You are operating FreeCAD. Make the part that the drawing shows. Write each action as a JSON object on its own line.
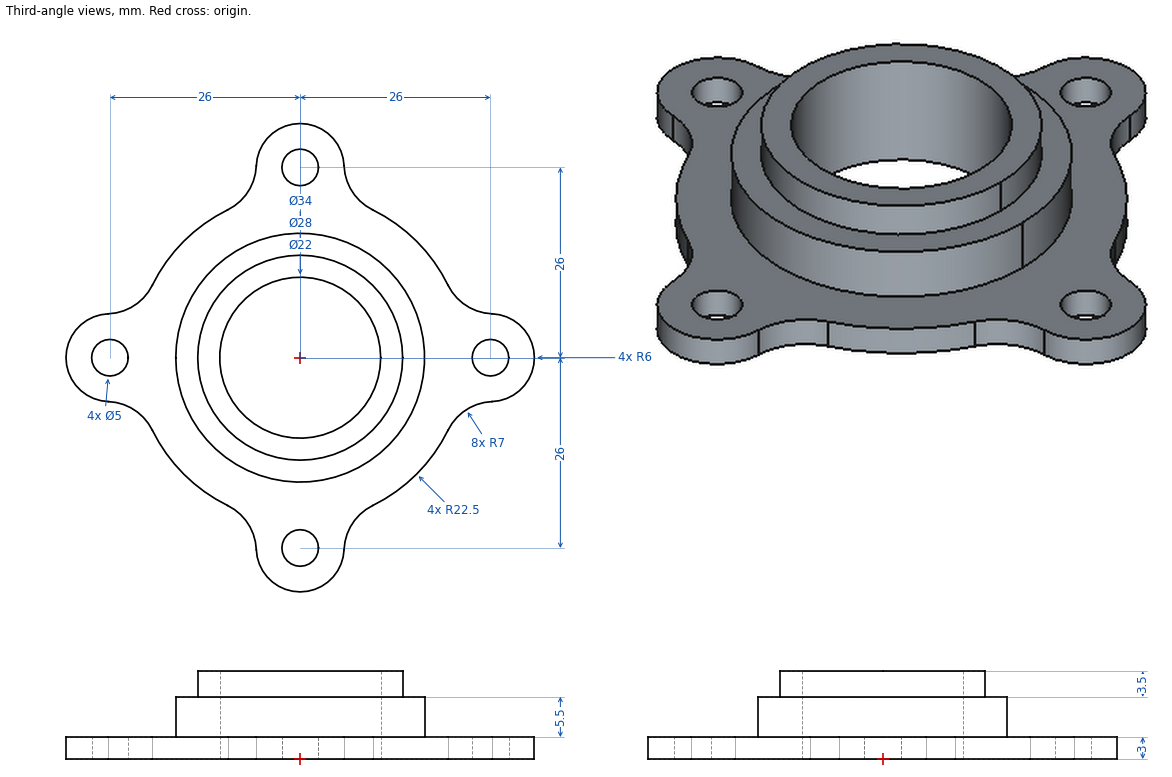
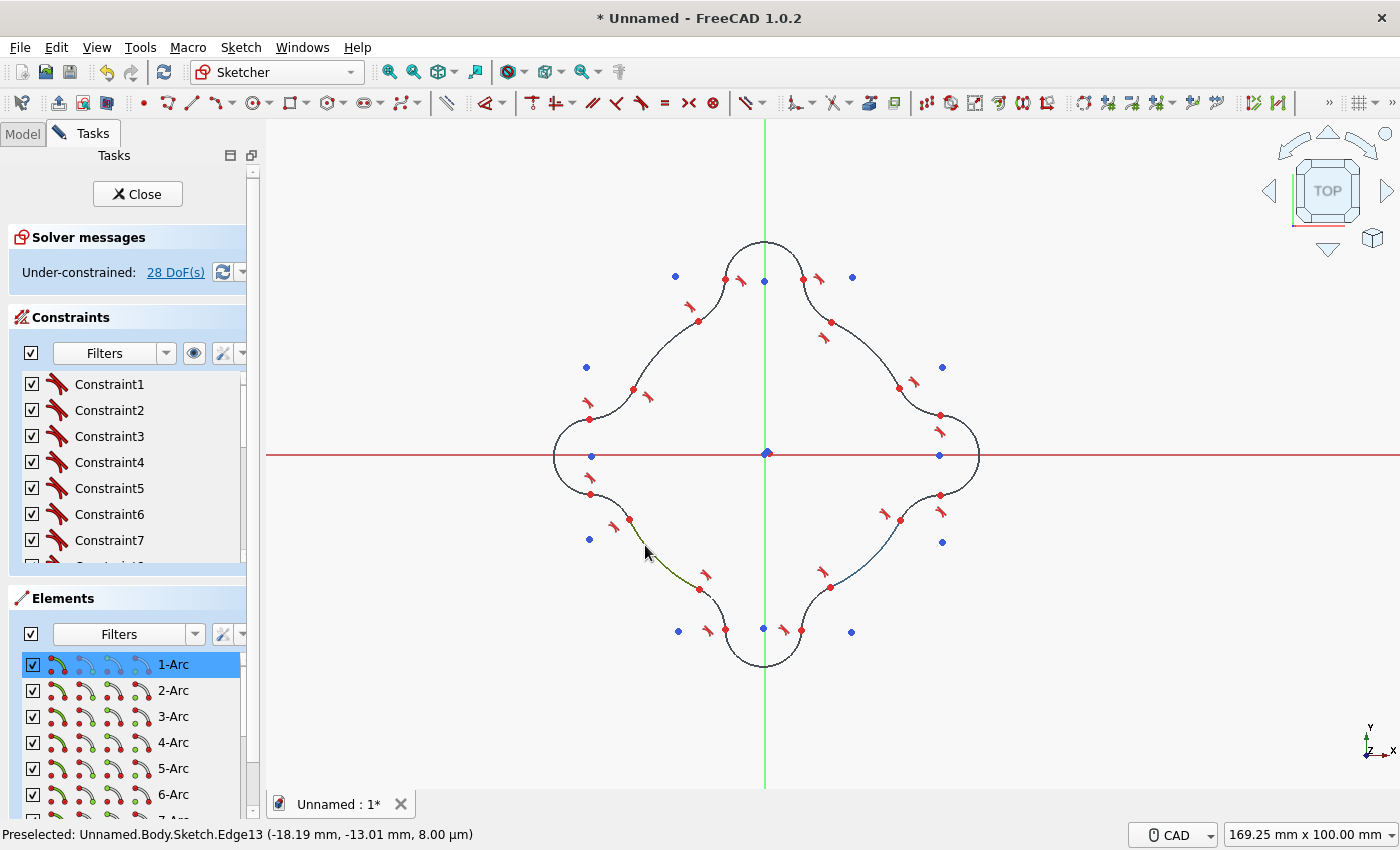
{"action": "left_click", "coordinate": [532, 104]}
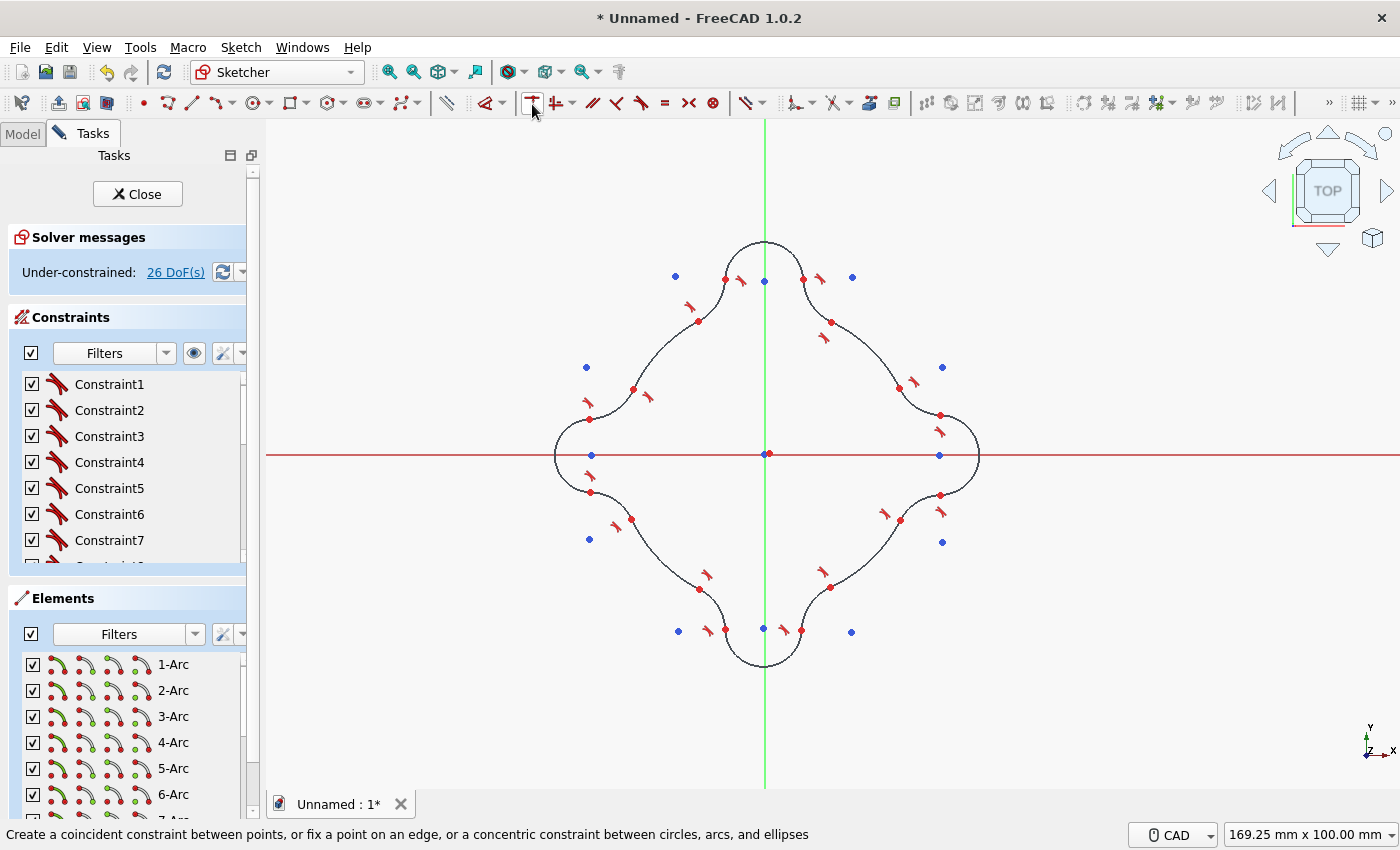
{"action": "left_click_drag", "start_coordinate": [755, 444], "coordinate": [780, 465]}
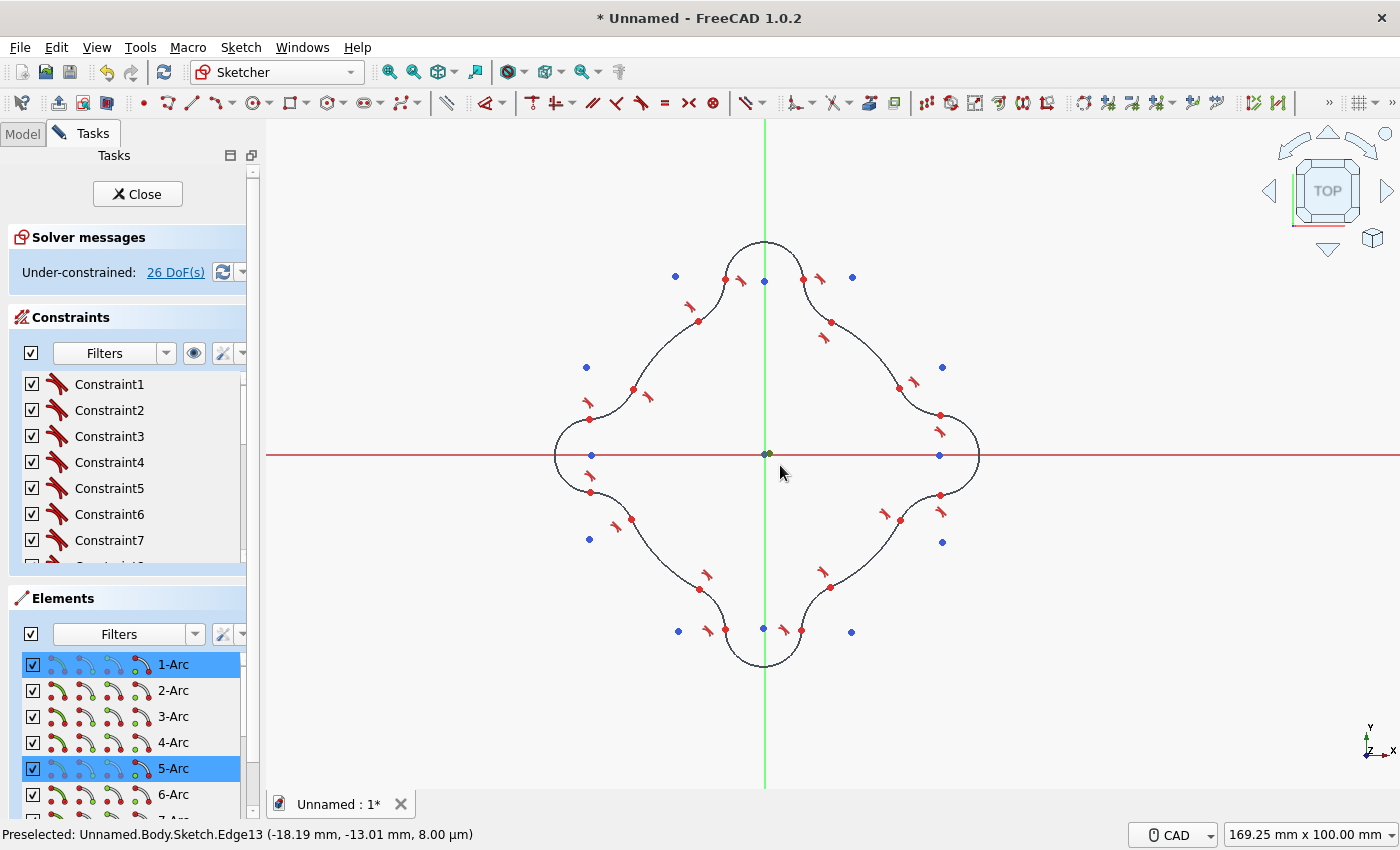
{"action": "left_click", "coordinate": [532, 104]}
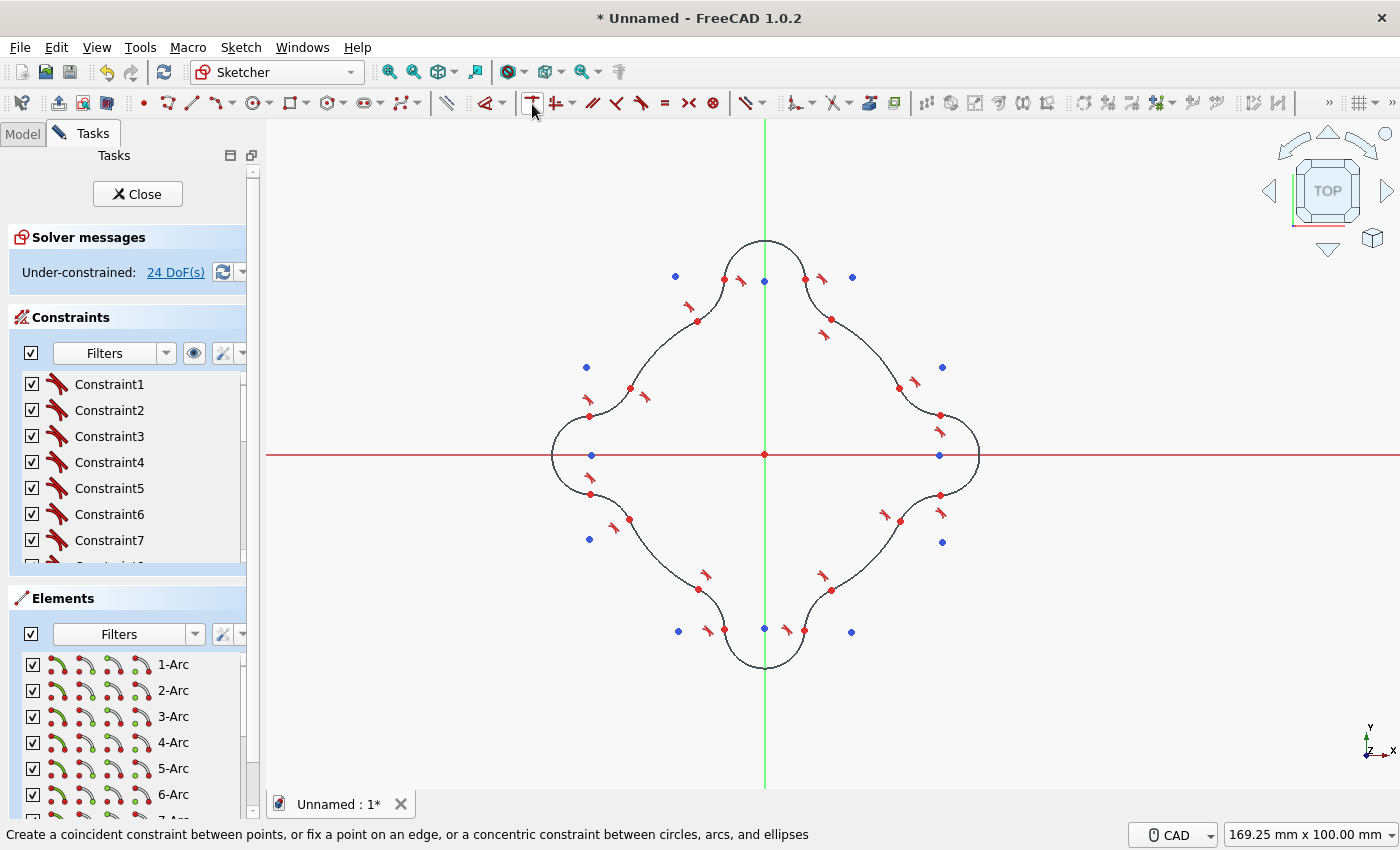
{"action": "left_click", "coordinate": [926, 498]}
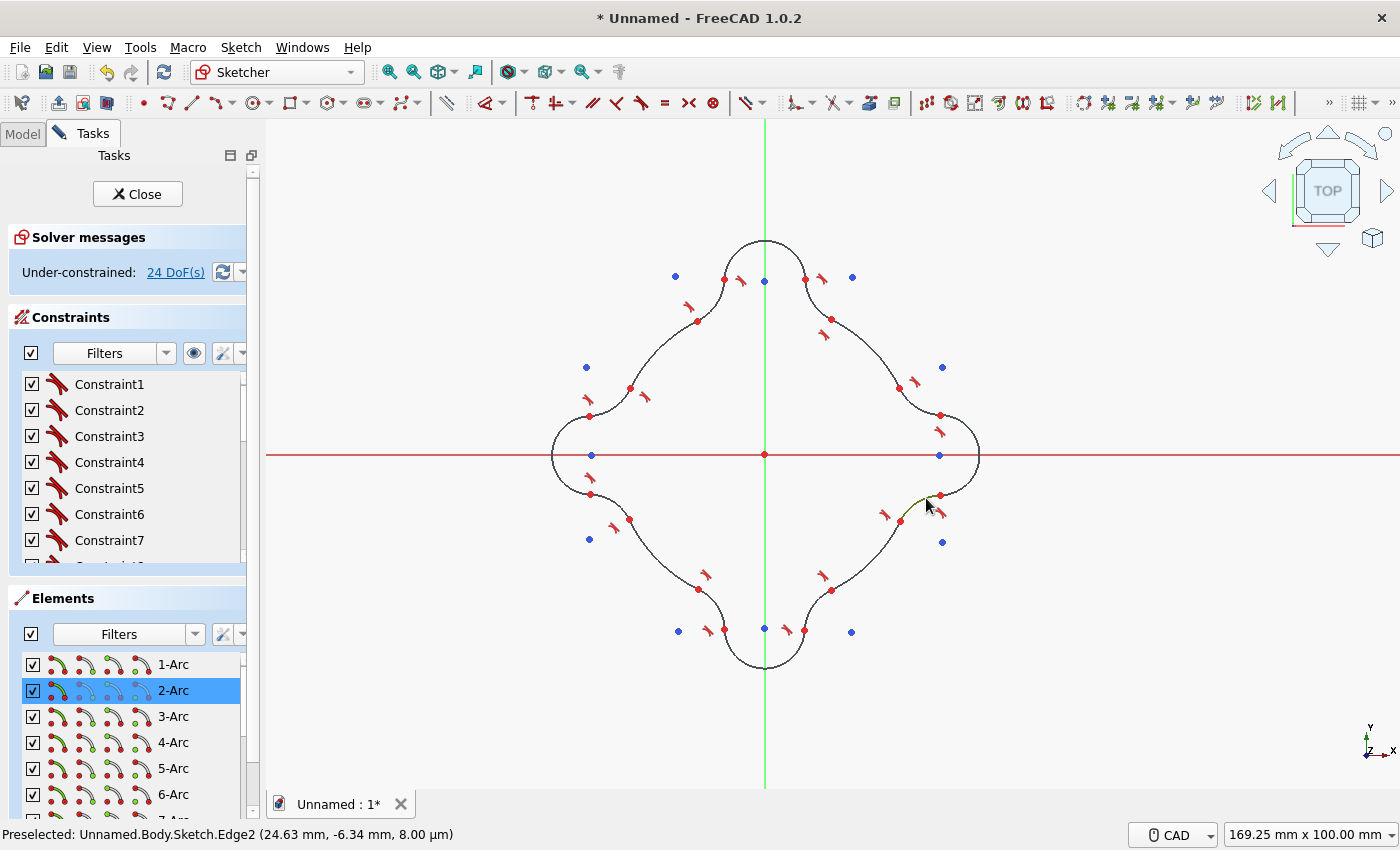
{"action": "left_click", "coordinate": [909, 401]}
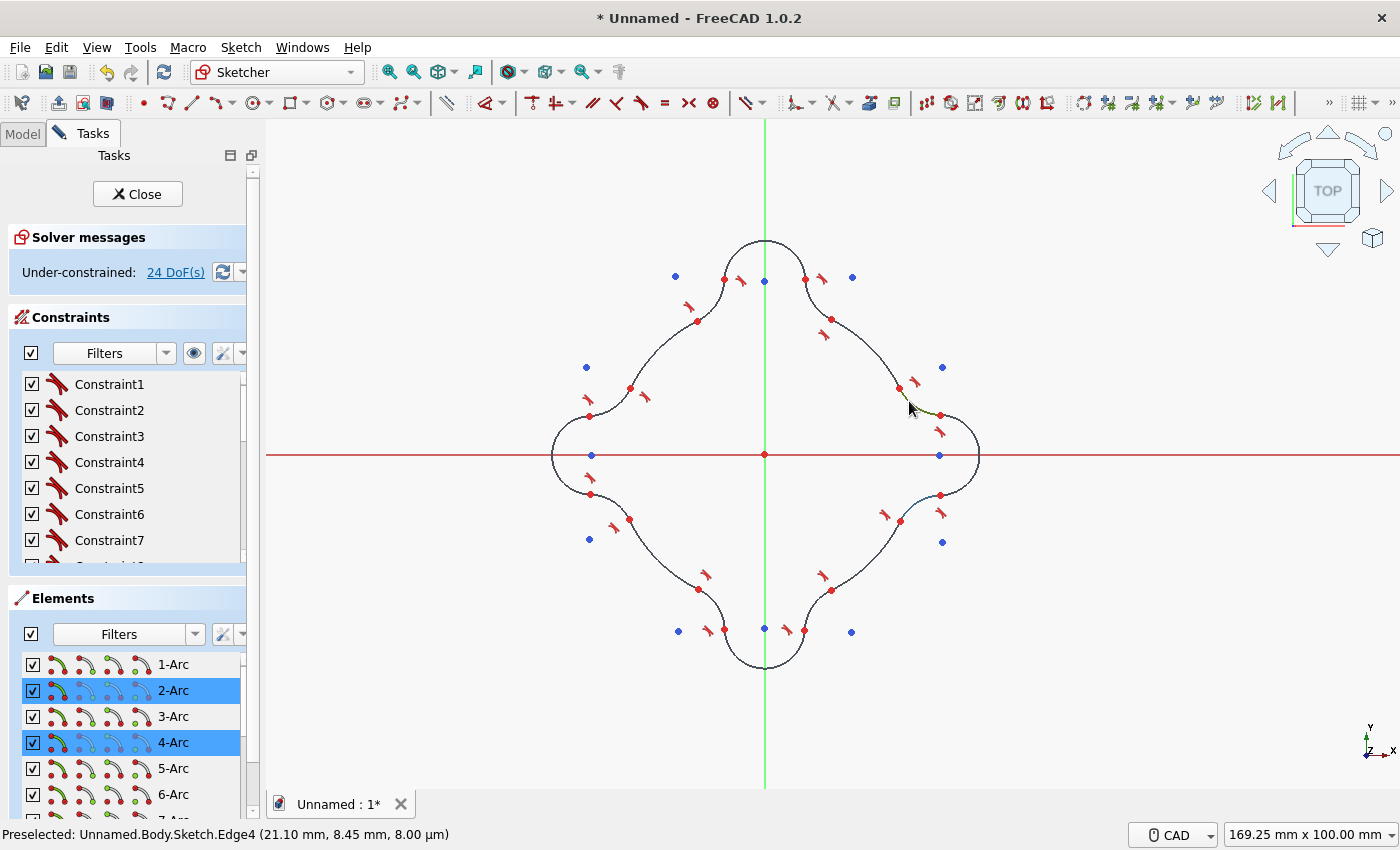
{"action": "left_click", "coordinate": [808, 294]}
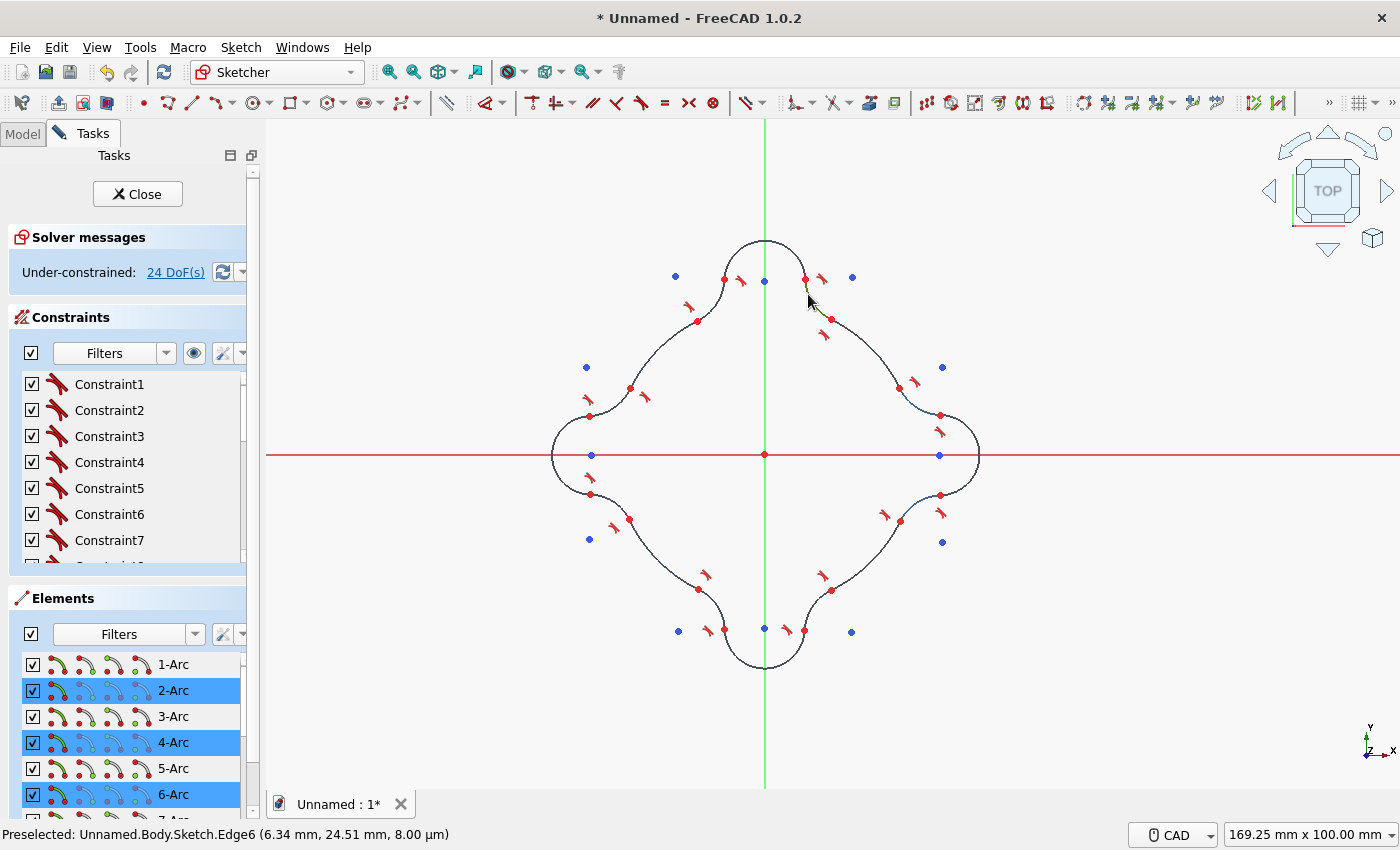
{"action": "left_click", "coordinate": [710, 312]}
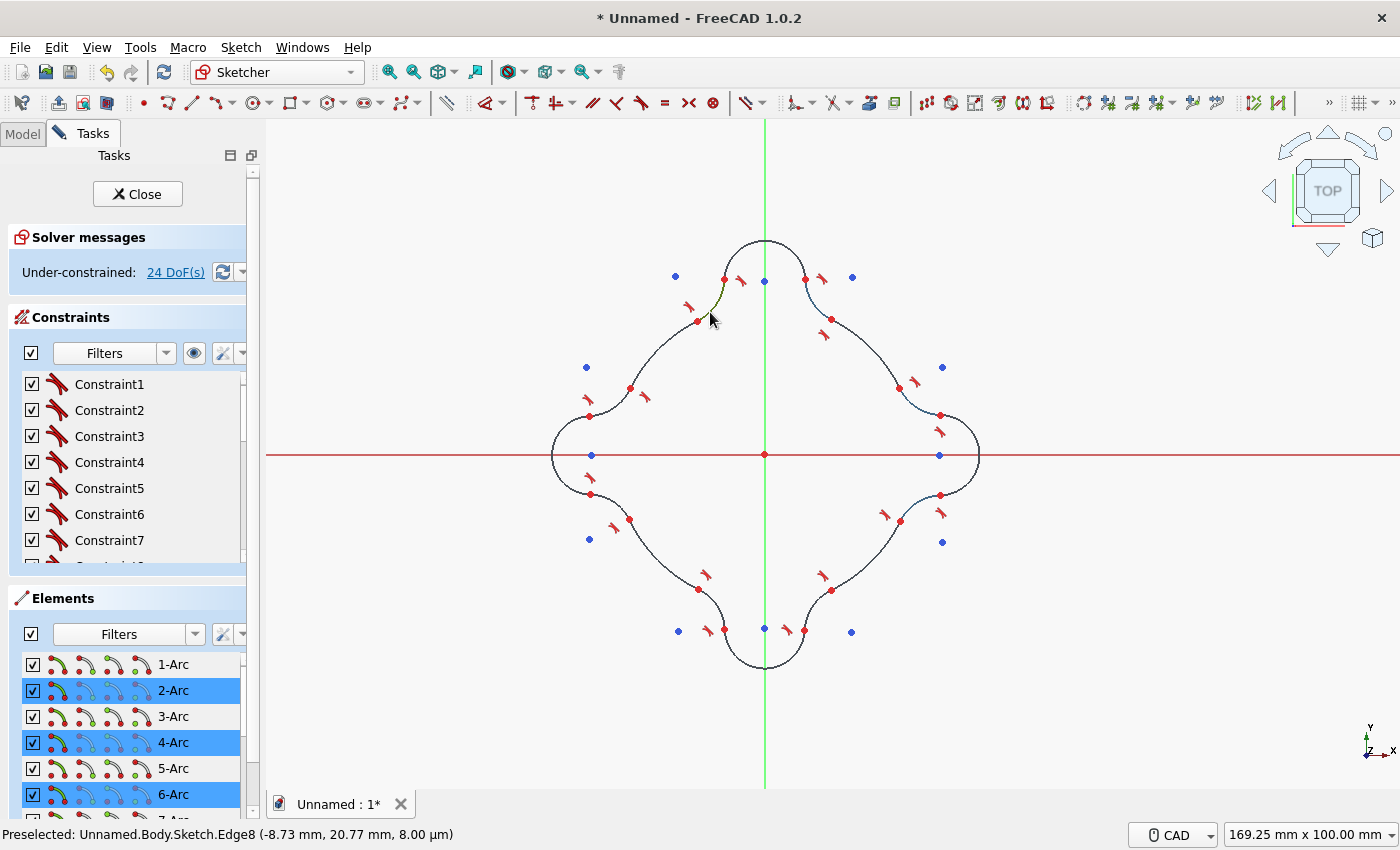
{"action": "left_click", "coordinate": [604, 413]}